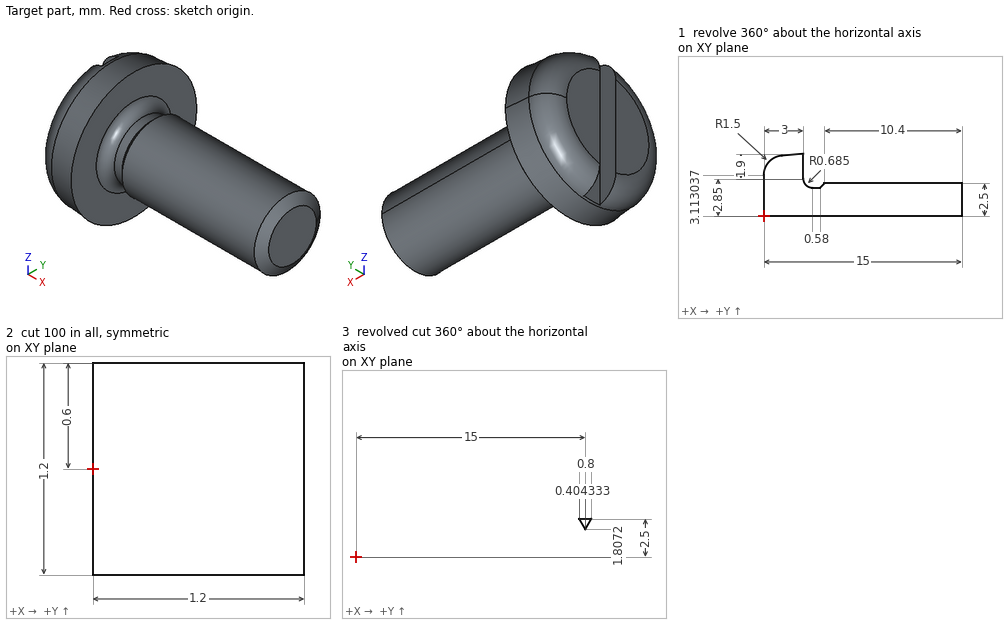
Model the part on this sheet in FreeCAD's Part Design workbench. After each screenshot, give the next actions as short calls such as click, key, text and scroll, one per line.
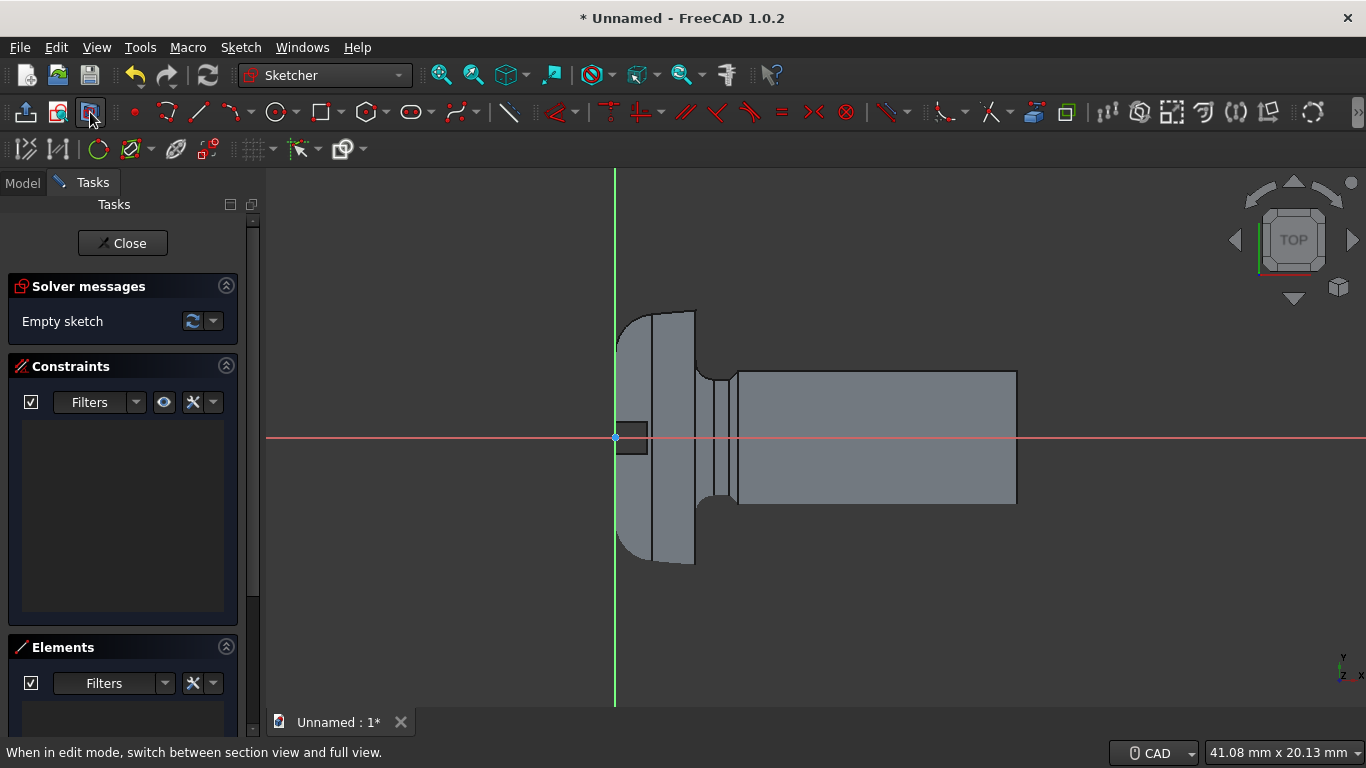
scroll(1031, 377, up, 15)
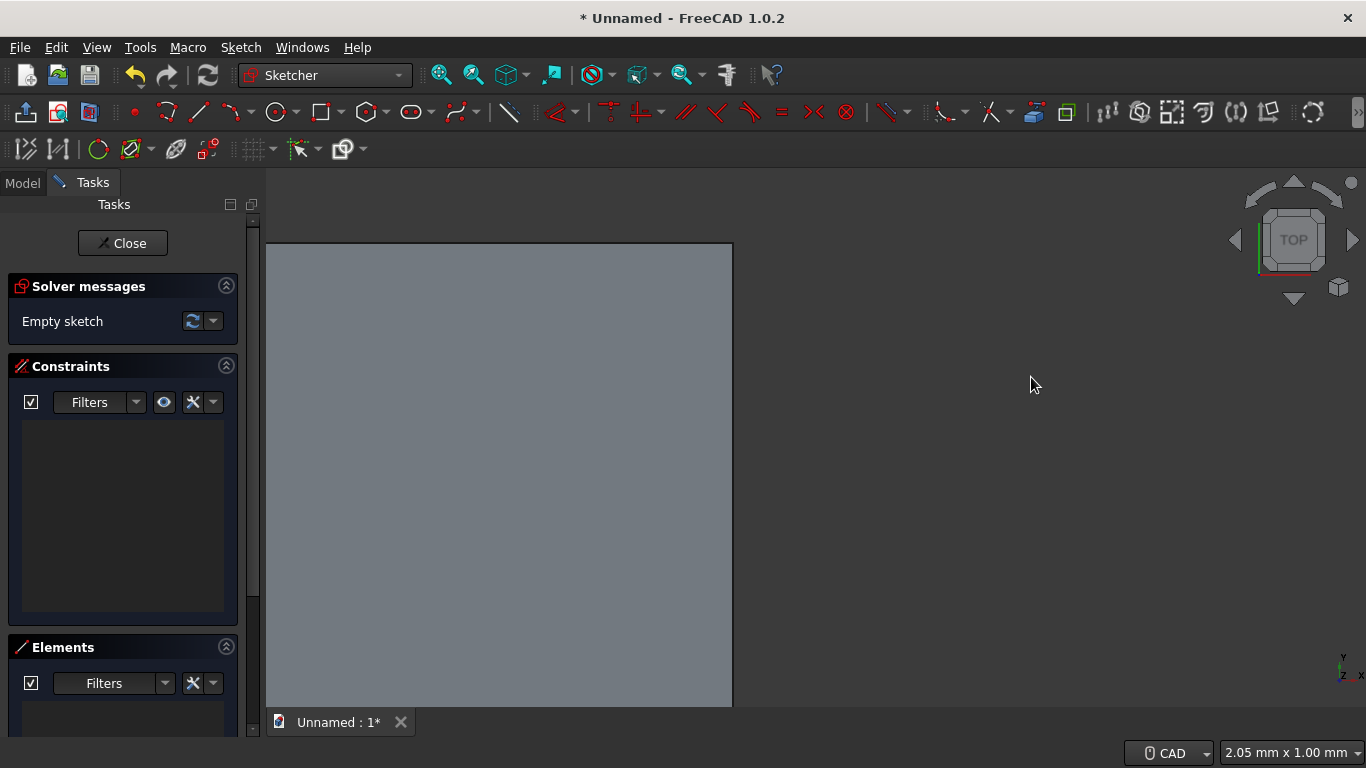
key(g)
key(m)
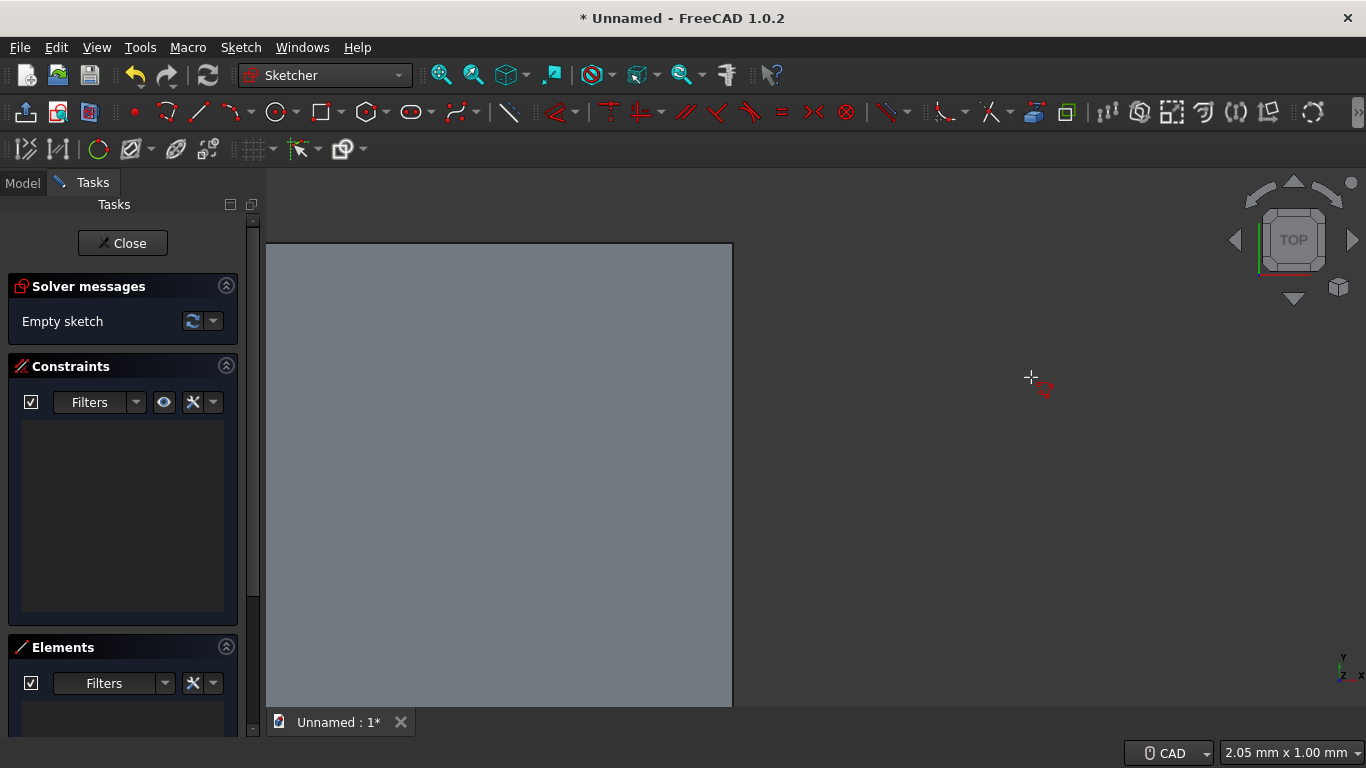
click(516, 243)
click(733, 616)
click(946, 243)
click(516, 244)
key(Escape)
key(Escape)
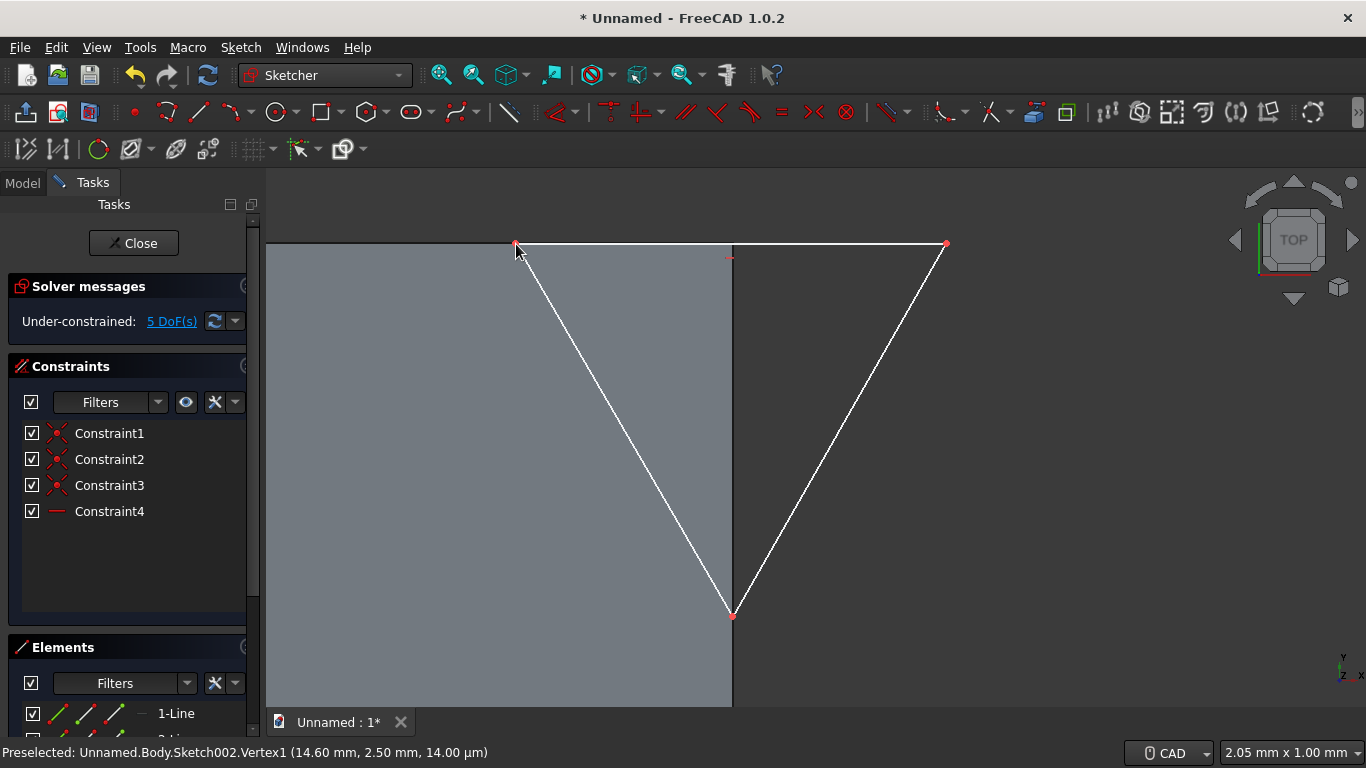
key(d)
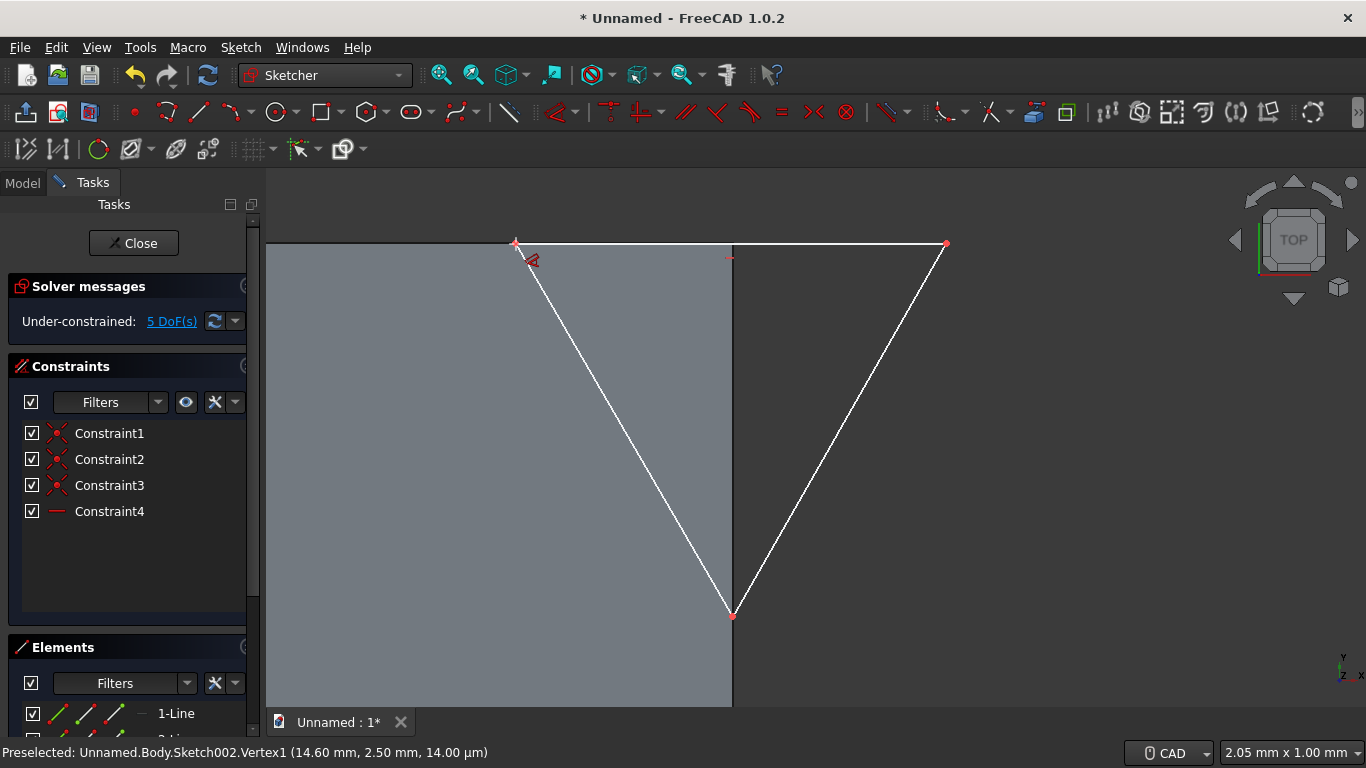
click(817, 244)
click(731, 210)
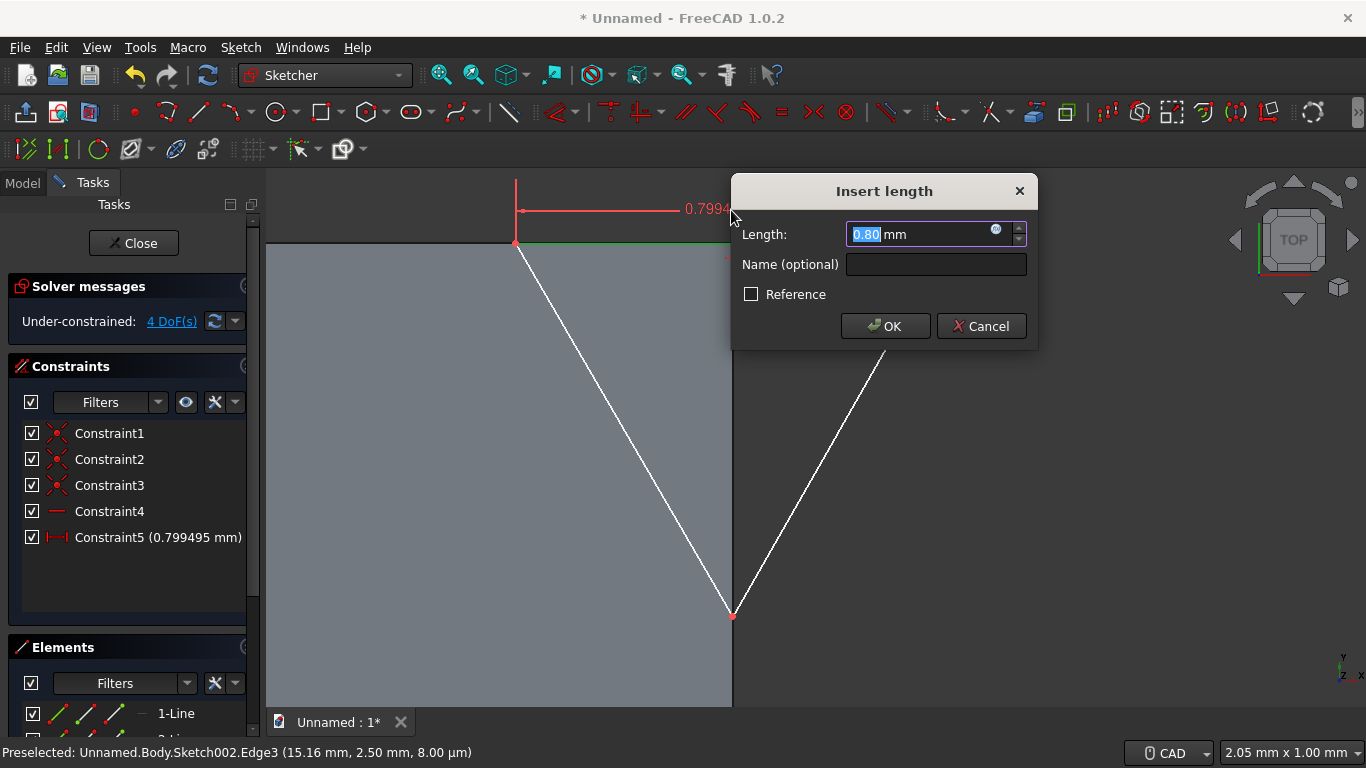
text(0.8)
key(Return)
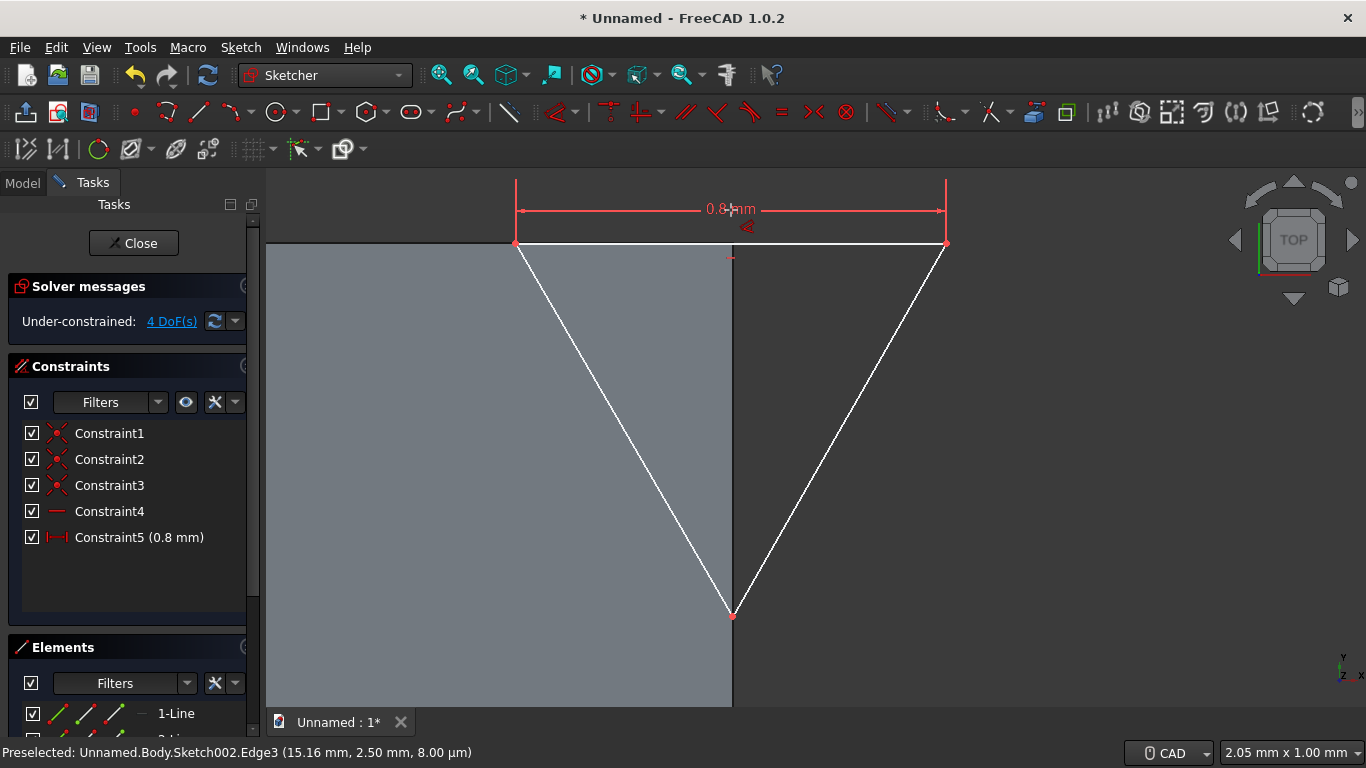
click(733, 617)
click(513, 583)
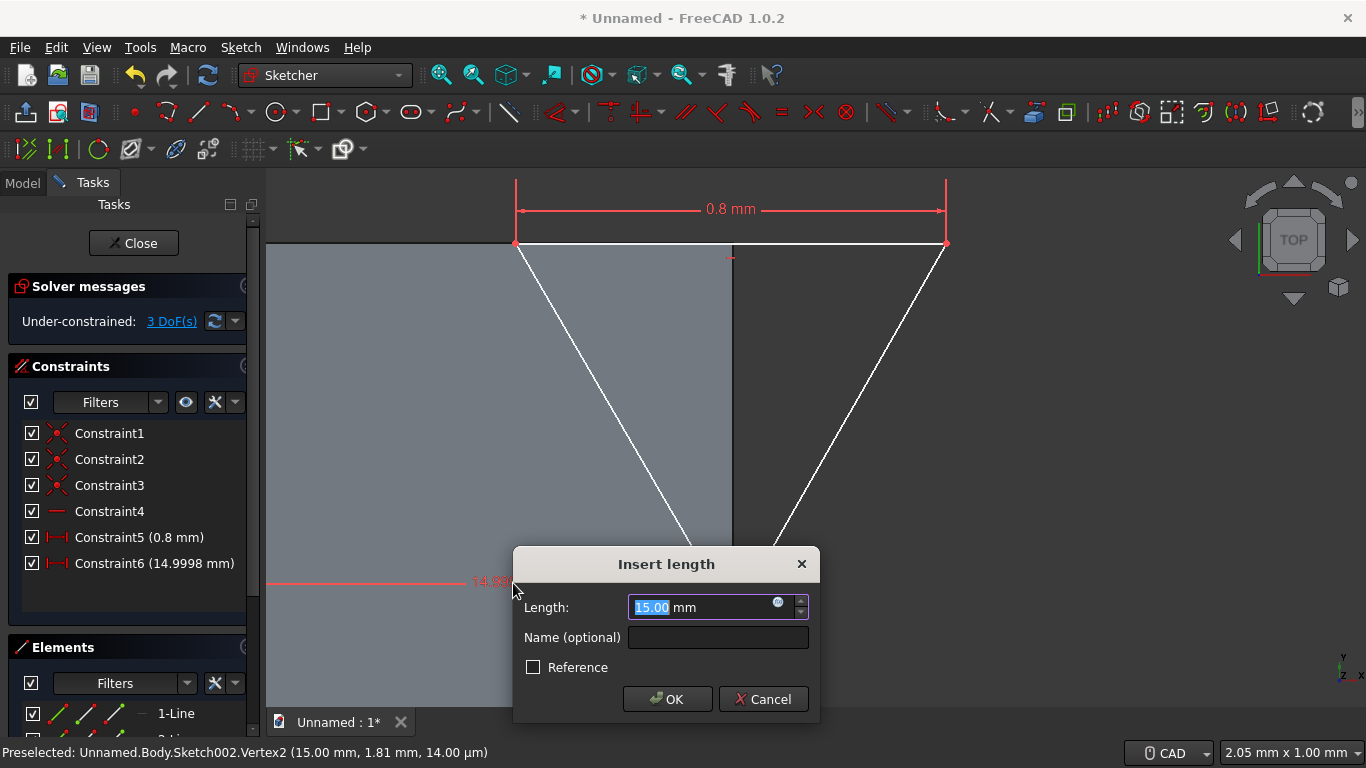
text(15)
key(Return)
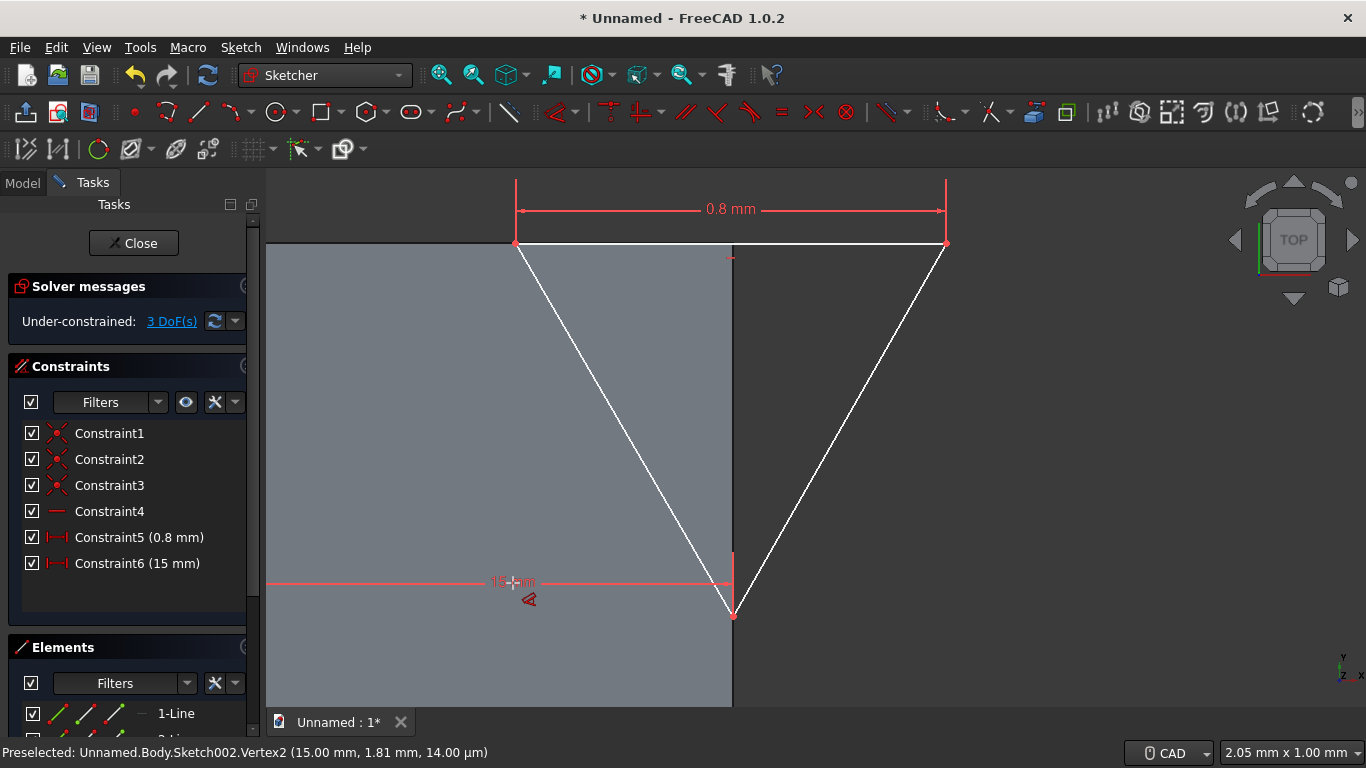
click(516, 244)
click(550, 461)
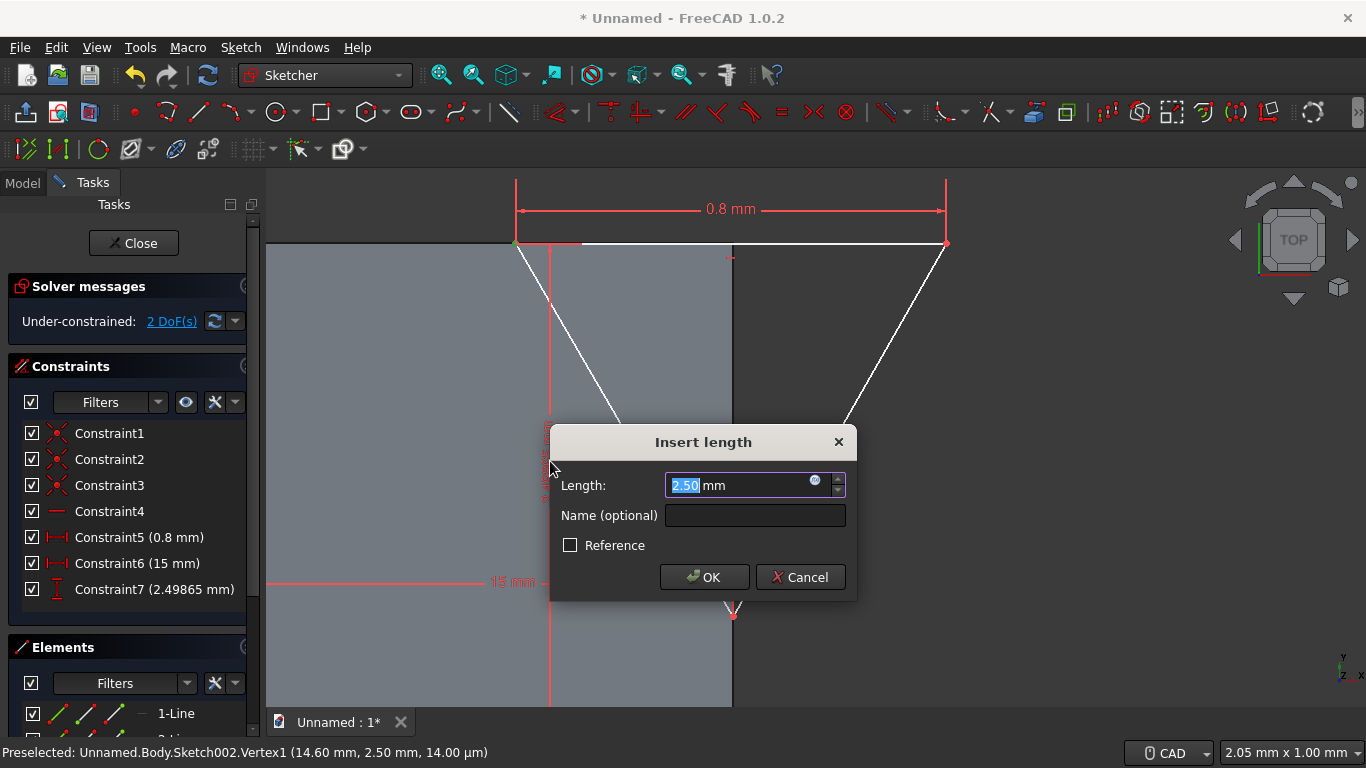
text(2.5)
key(Return)